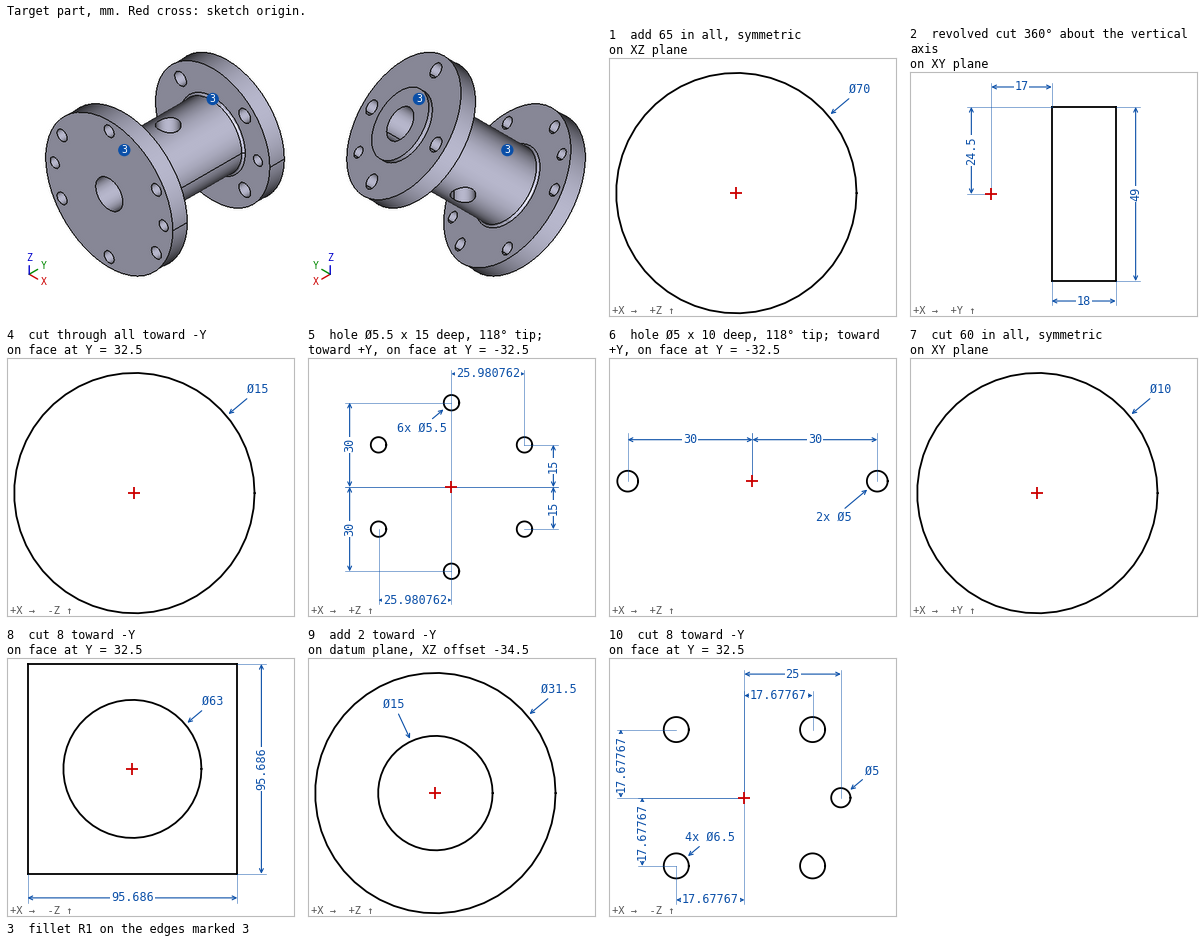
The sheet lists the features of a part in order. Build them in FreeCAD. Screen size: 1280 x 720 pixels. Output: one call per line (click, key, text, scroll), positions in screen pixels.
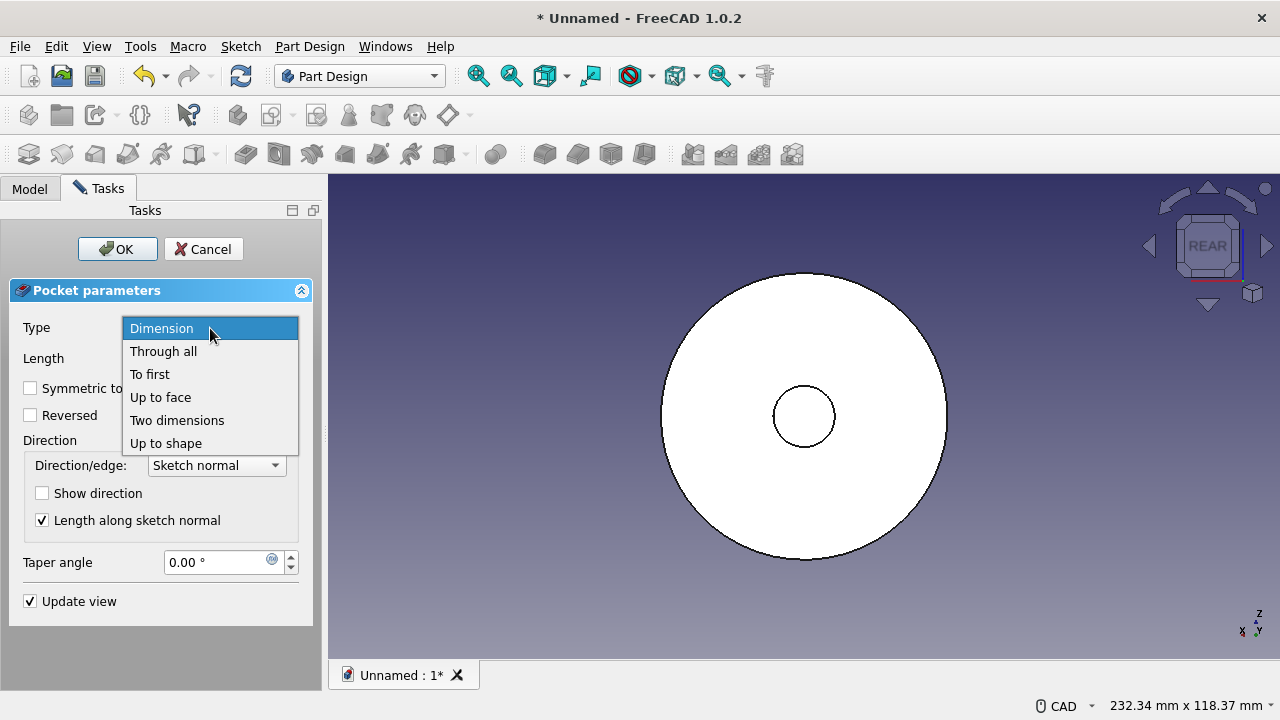
click(208, 352)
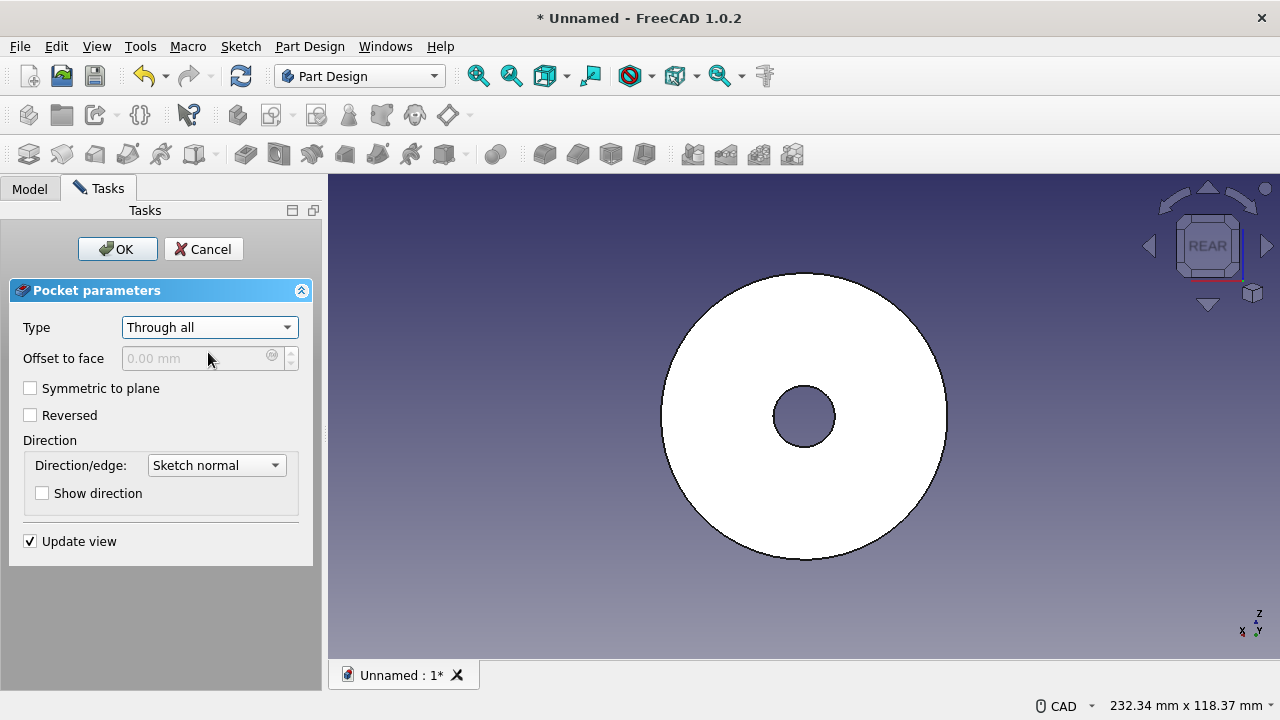
click(118, 249)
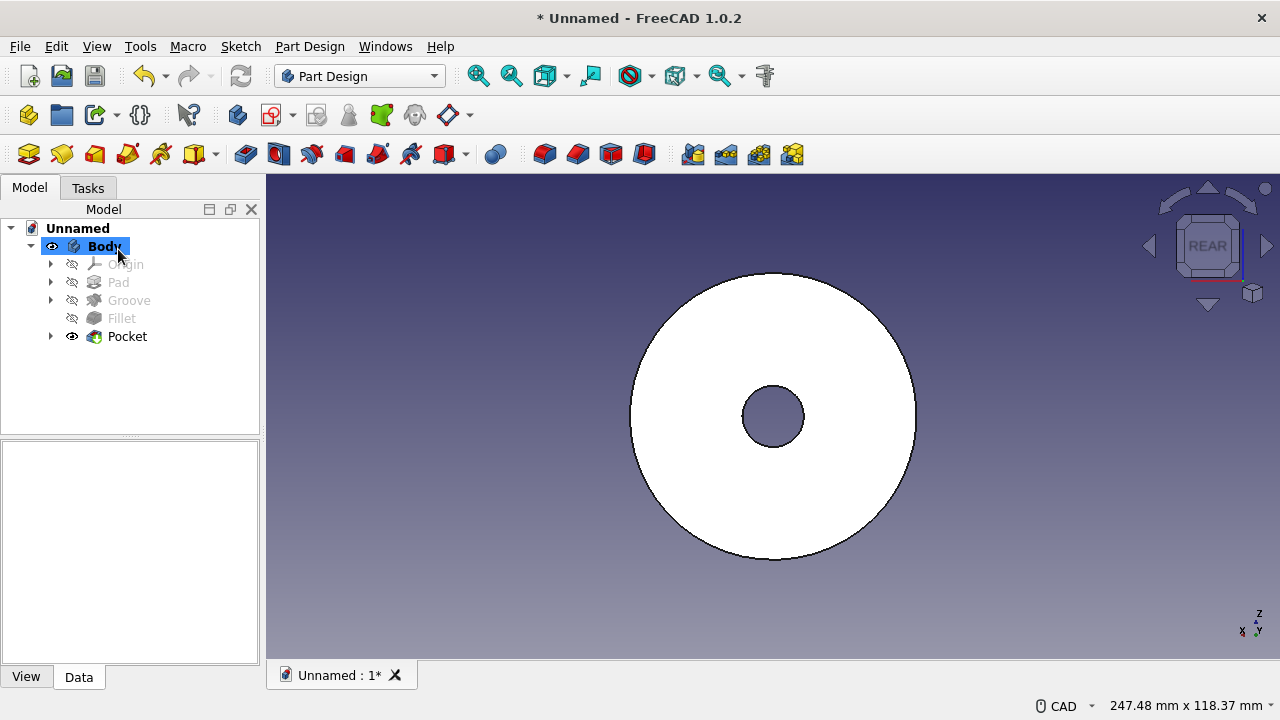
key(0)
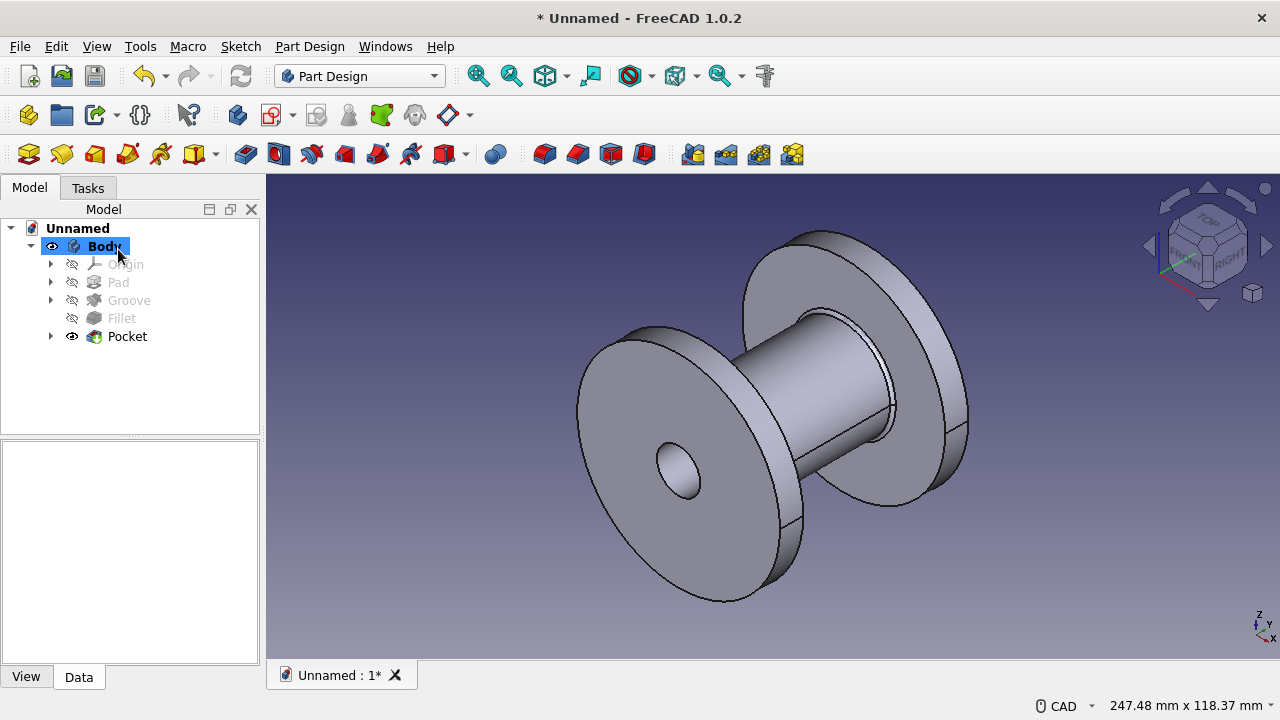
click(708, 553)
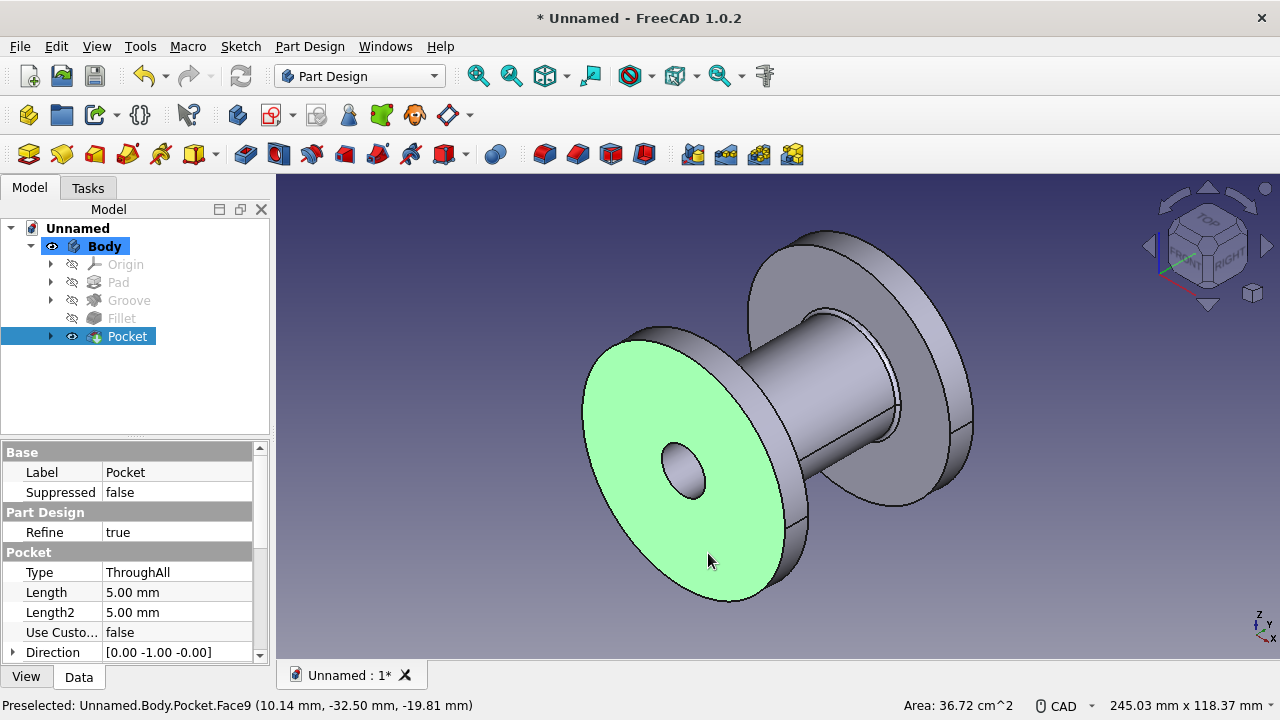
click(270, 116)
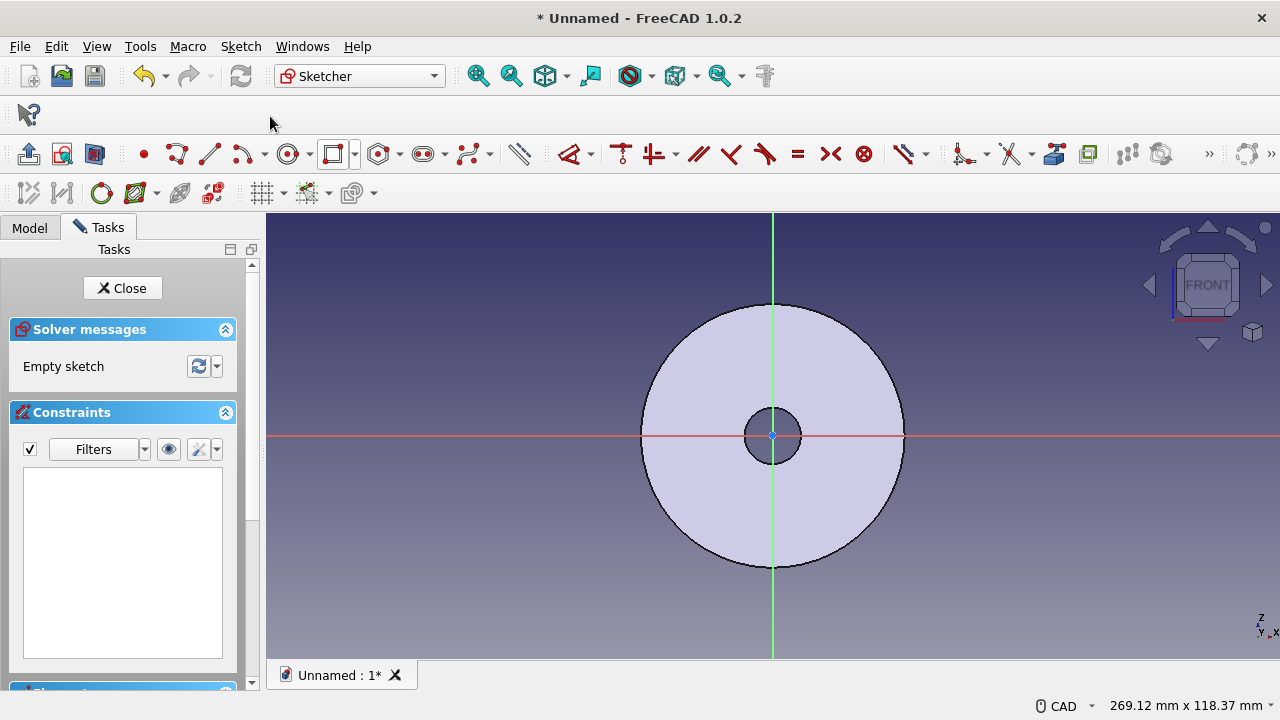
click(288, 154)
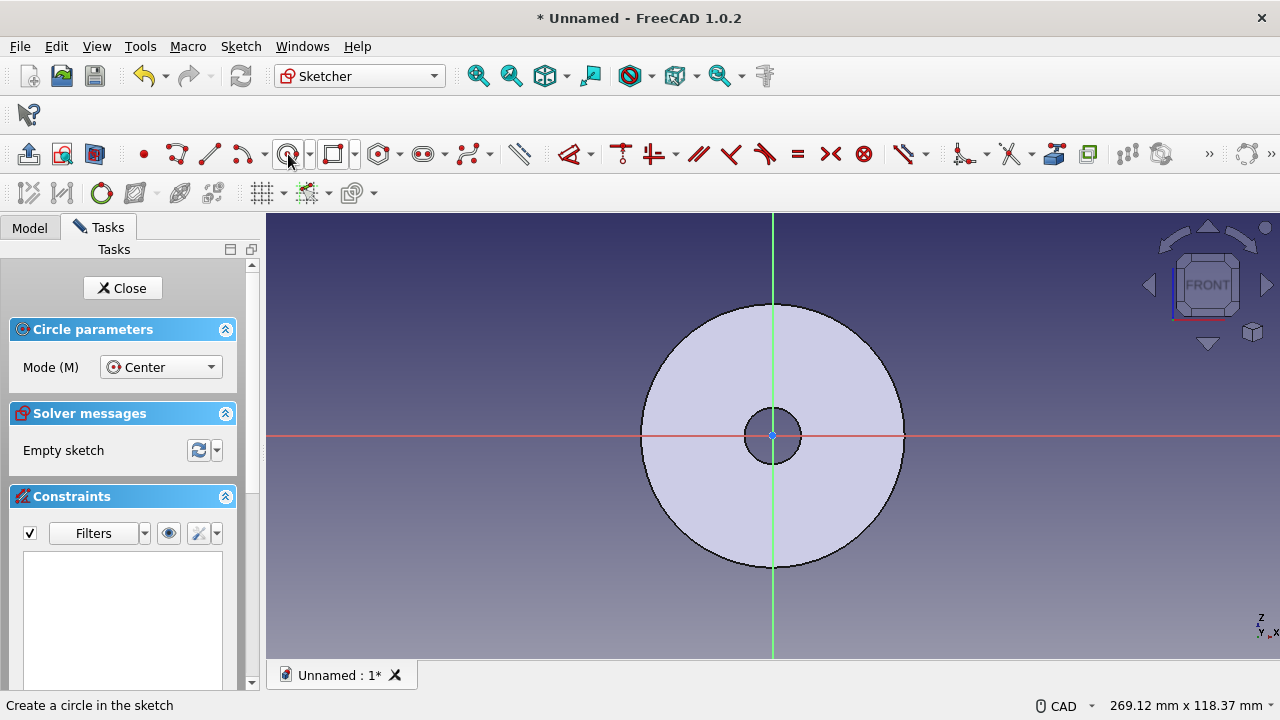
scroll(773, 323, up, 4)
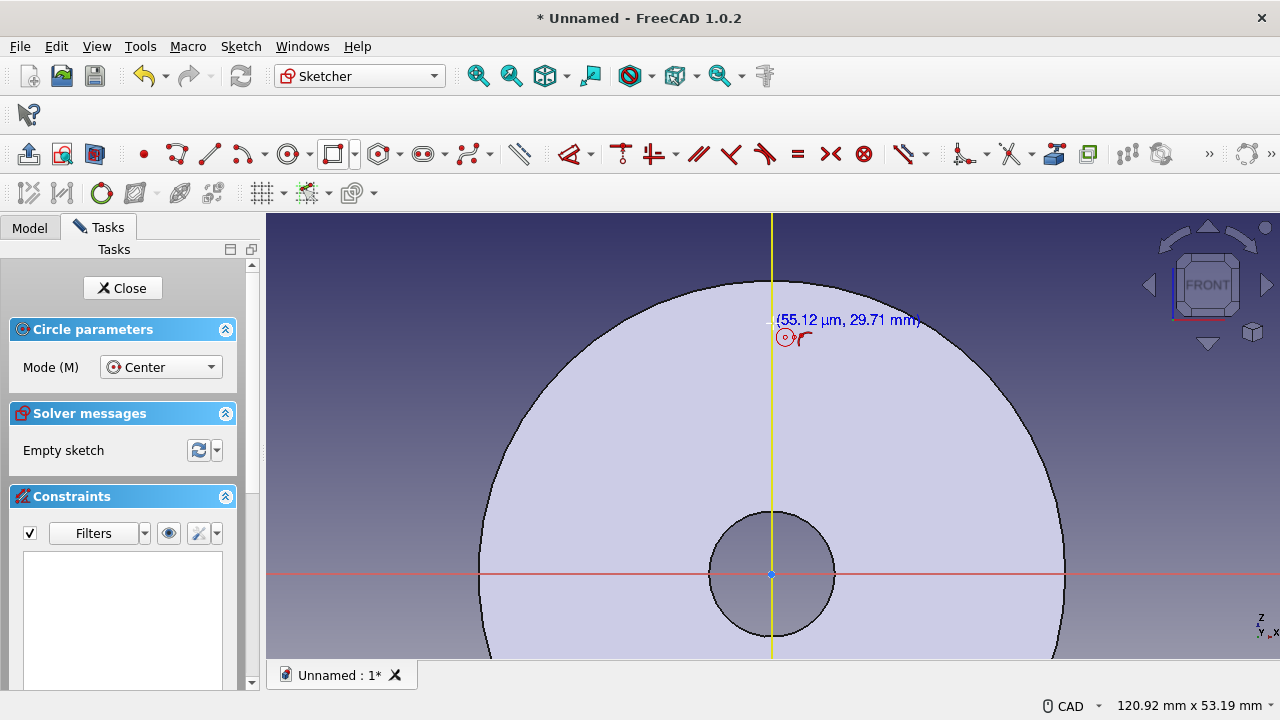
click(772, 322)
move(788, 306)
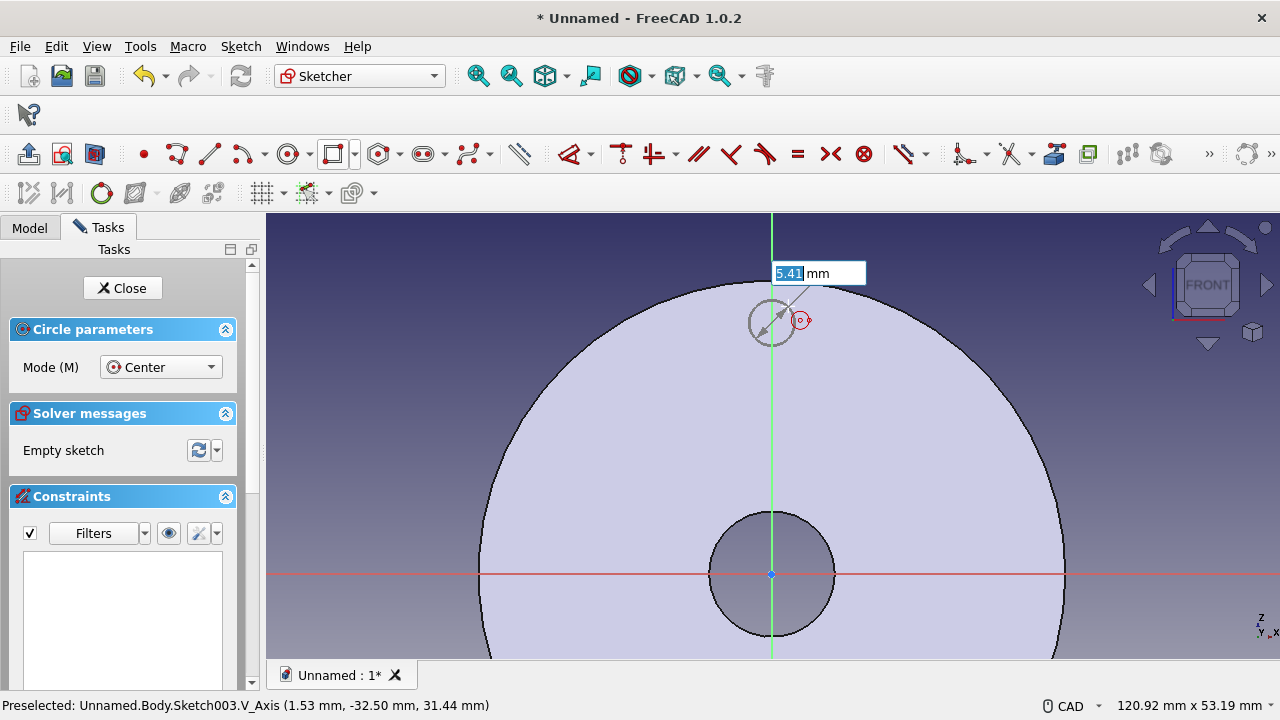
text(5.5)
key(Return)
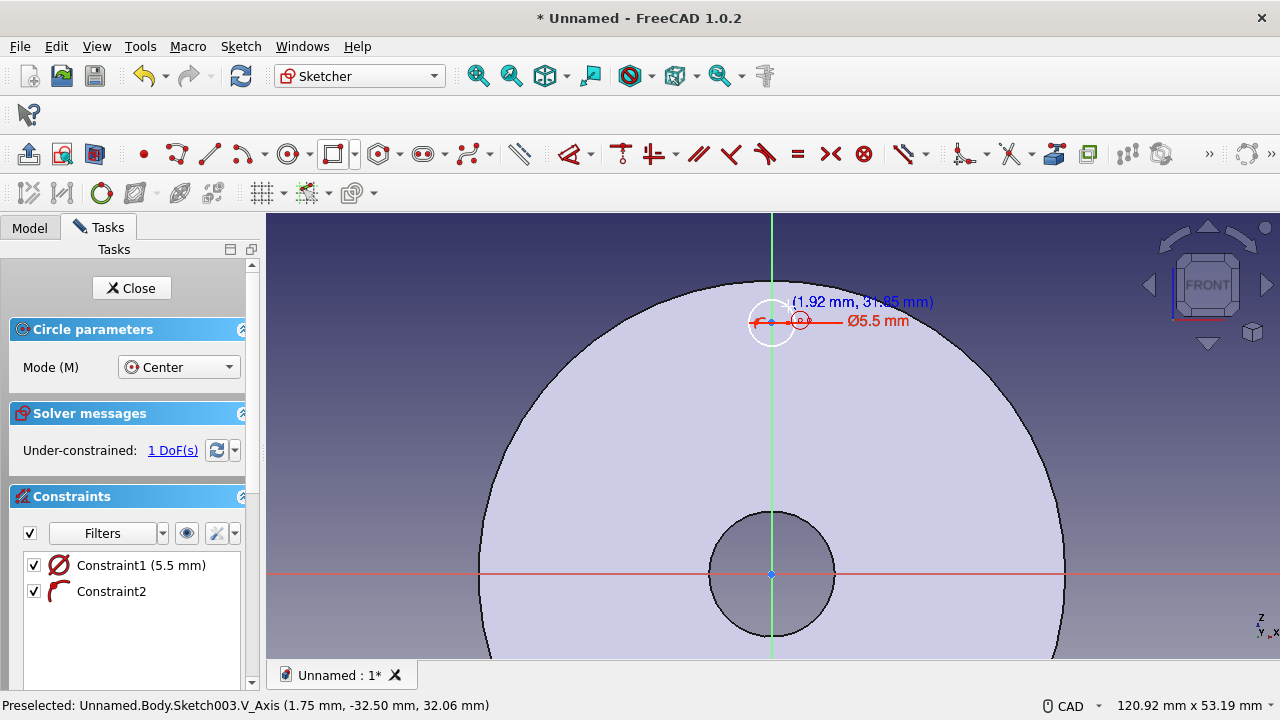
click(990, 448)
move(1006, 432)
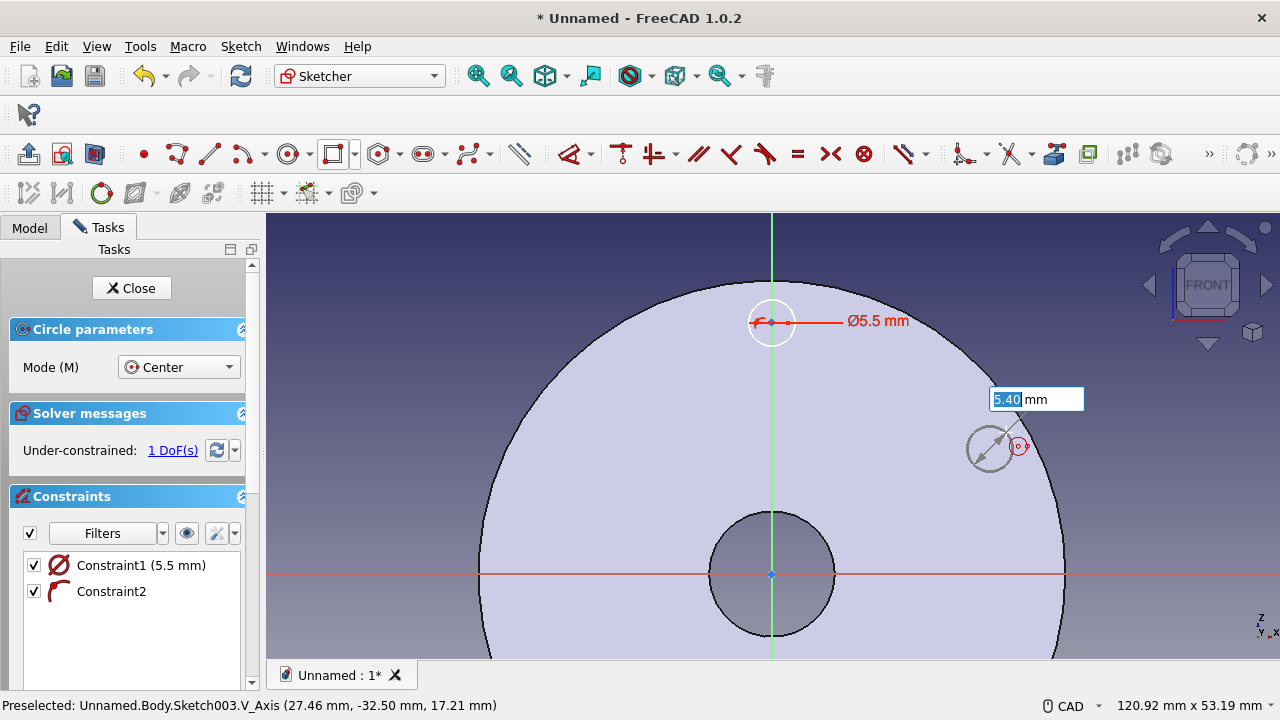
text(5.5)
key(Return)